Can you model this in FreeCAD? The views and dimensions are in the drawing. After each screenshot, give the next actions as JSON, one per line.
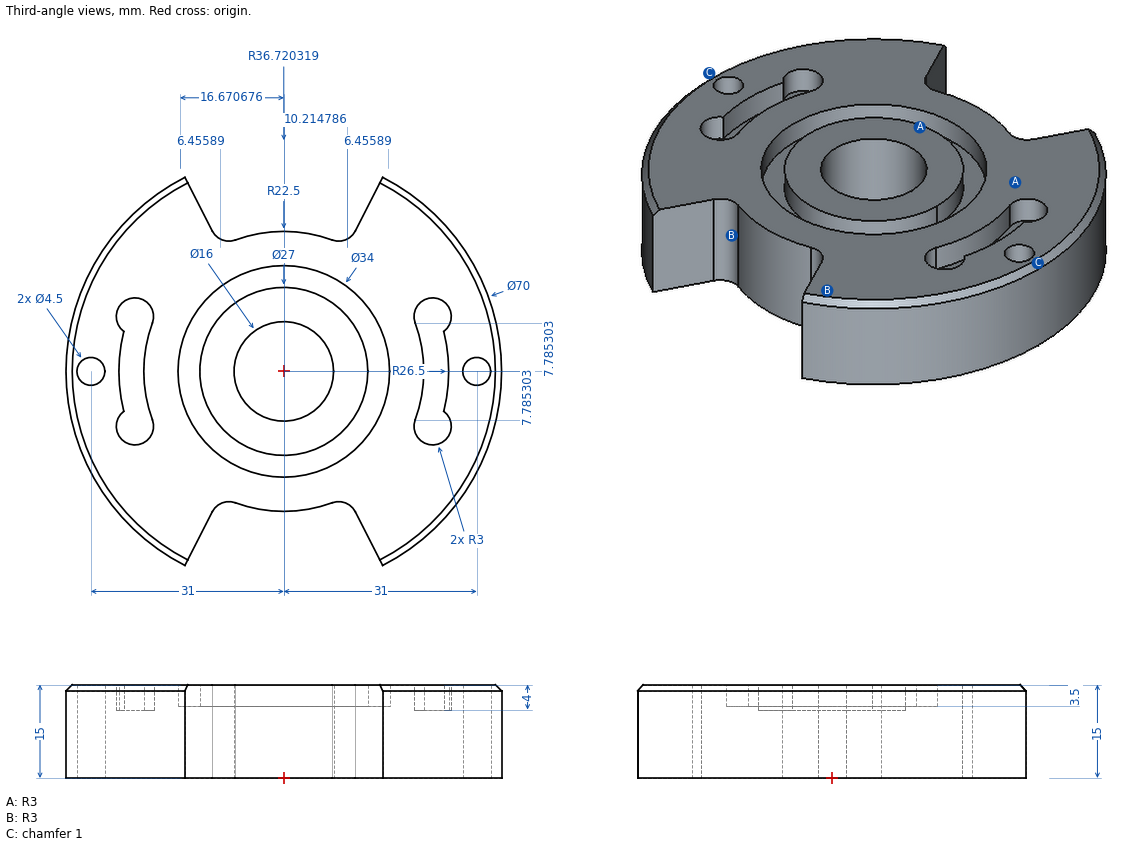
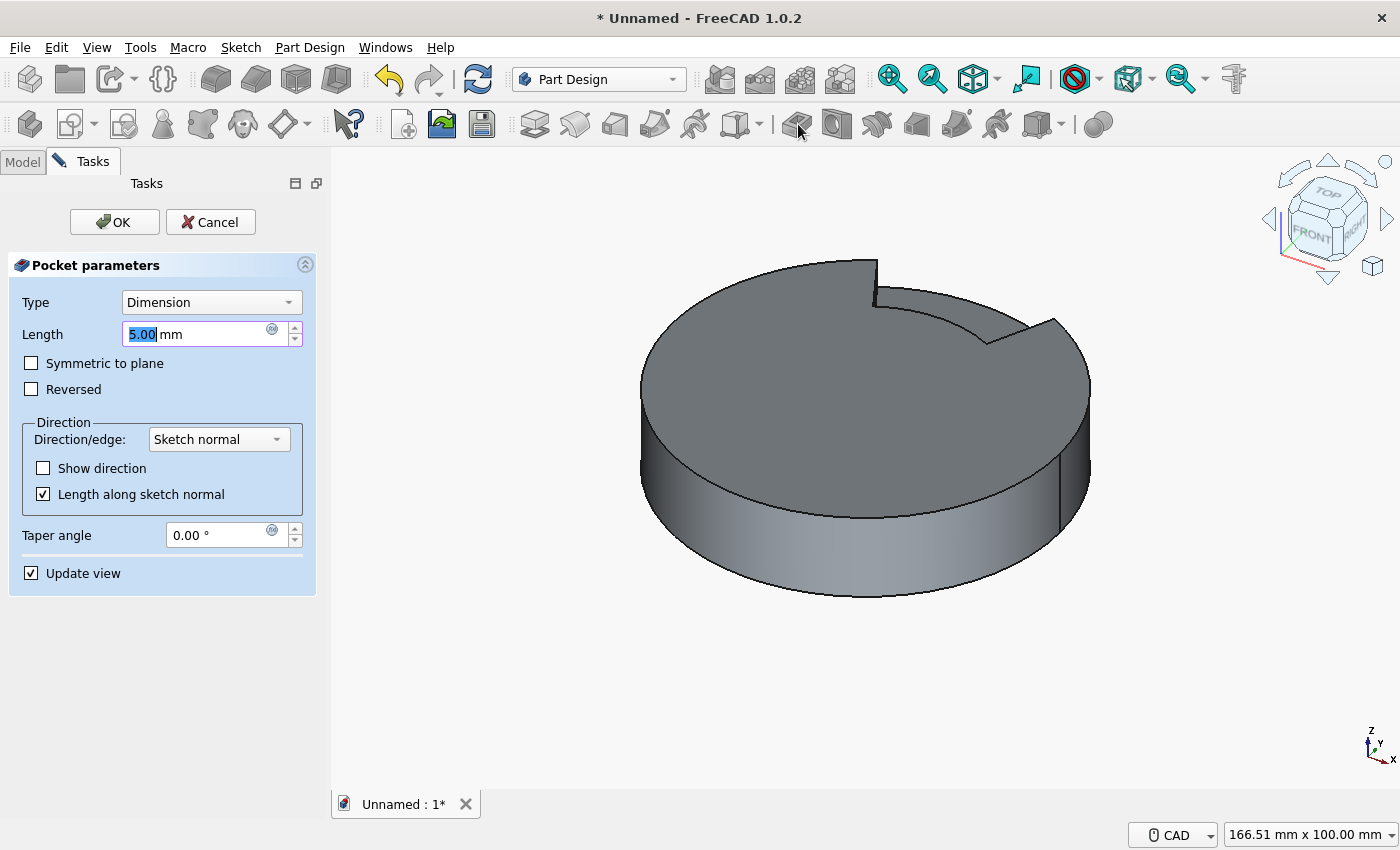
{"action": "type", "text": "15"}
{"action": "key", "text": "Tab"}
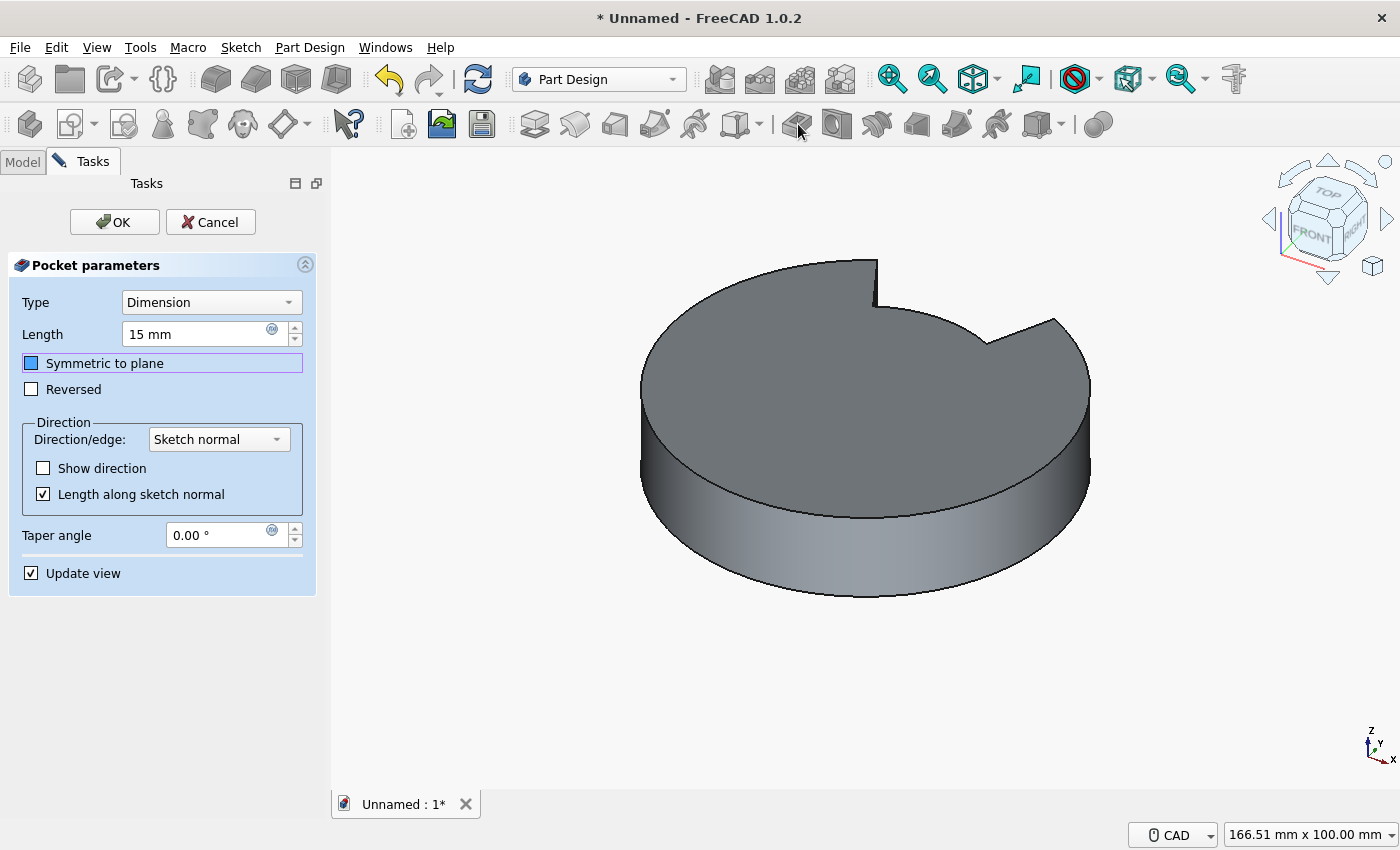
{"action": "left_click", "coordinate": [115, 222]}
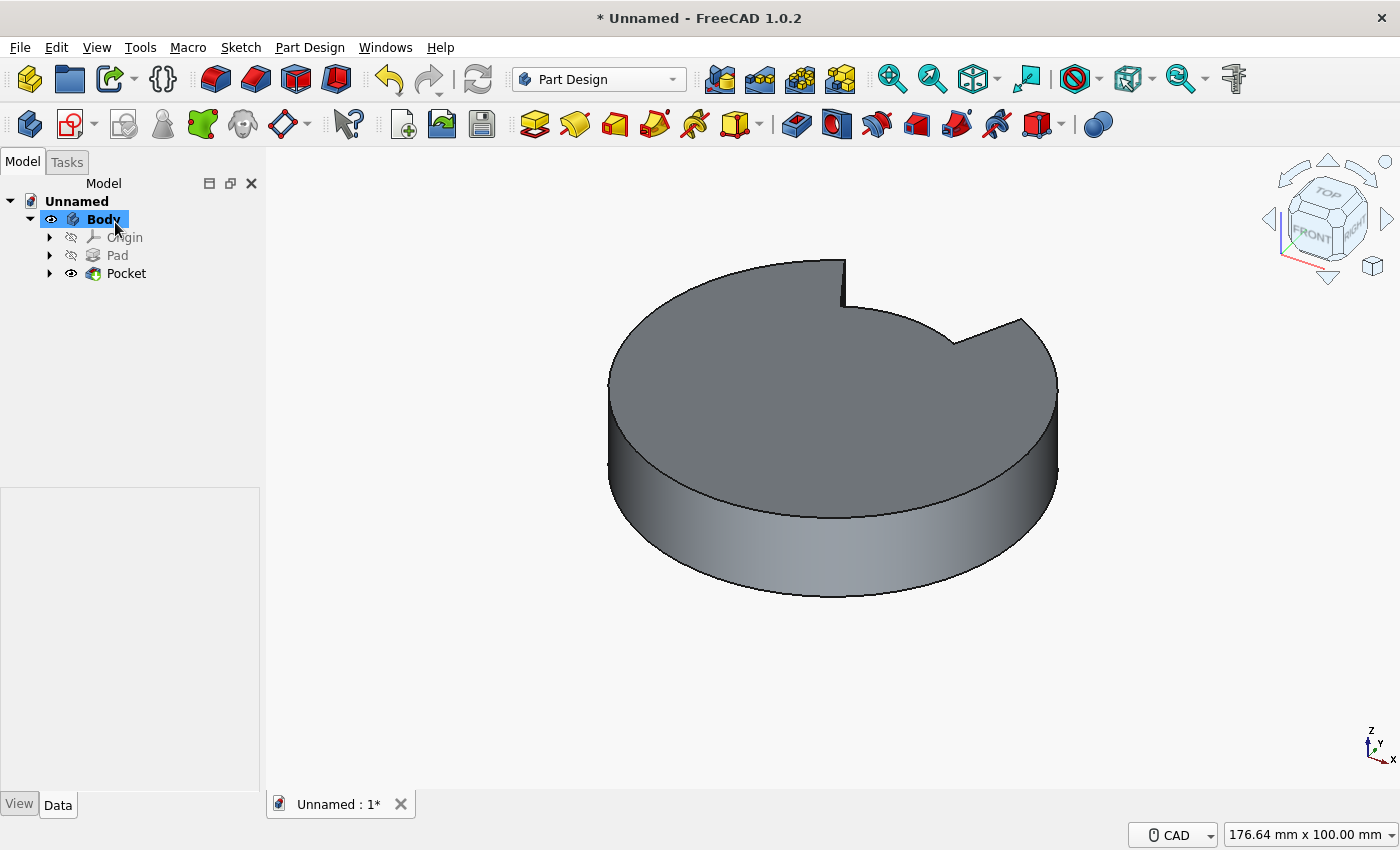
{"action": "key", "text": "0"}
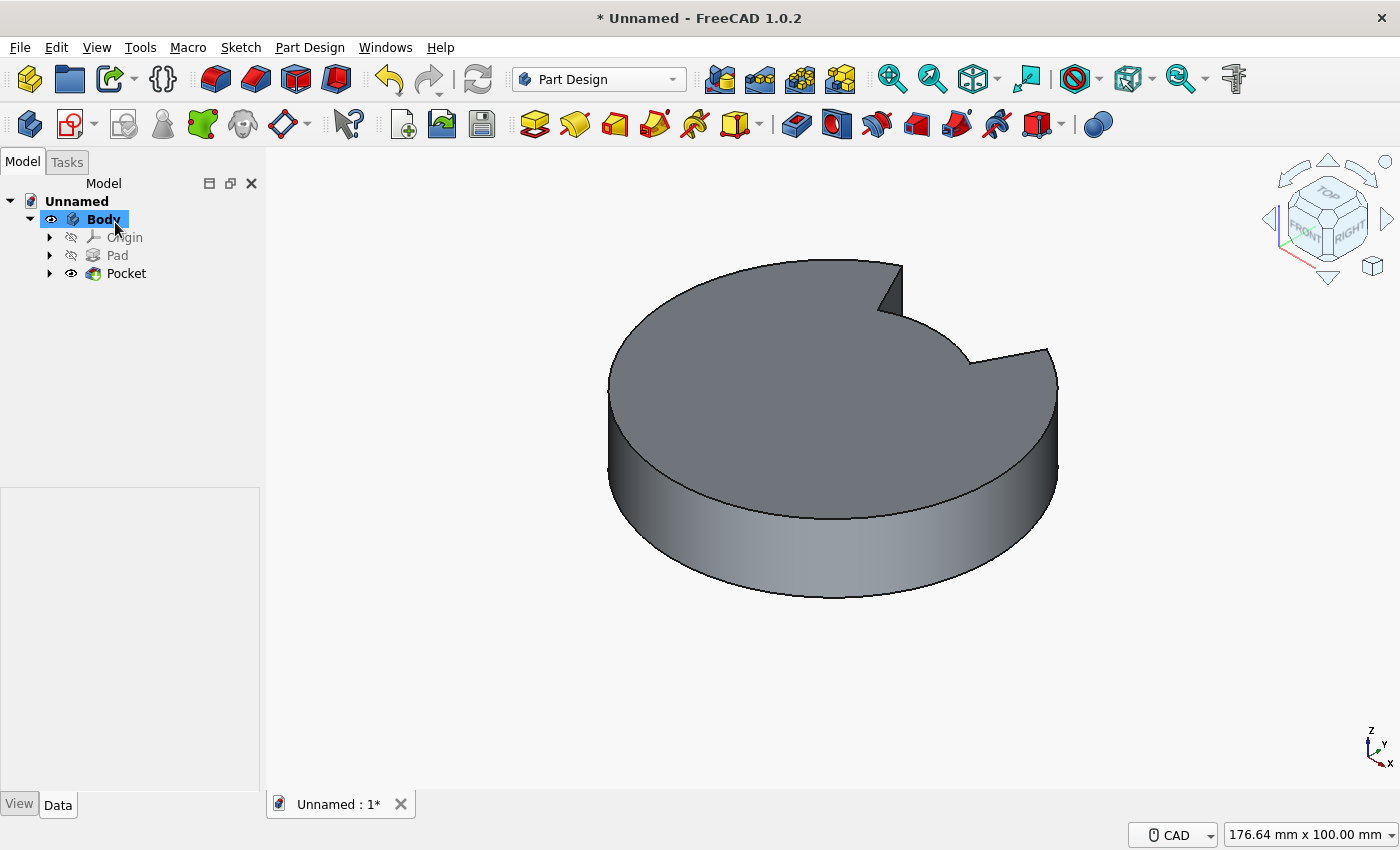
{"action": "key", "text": "2"}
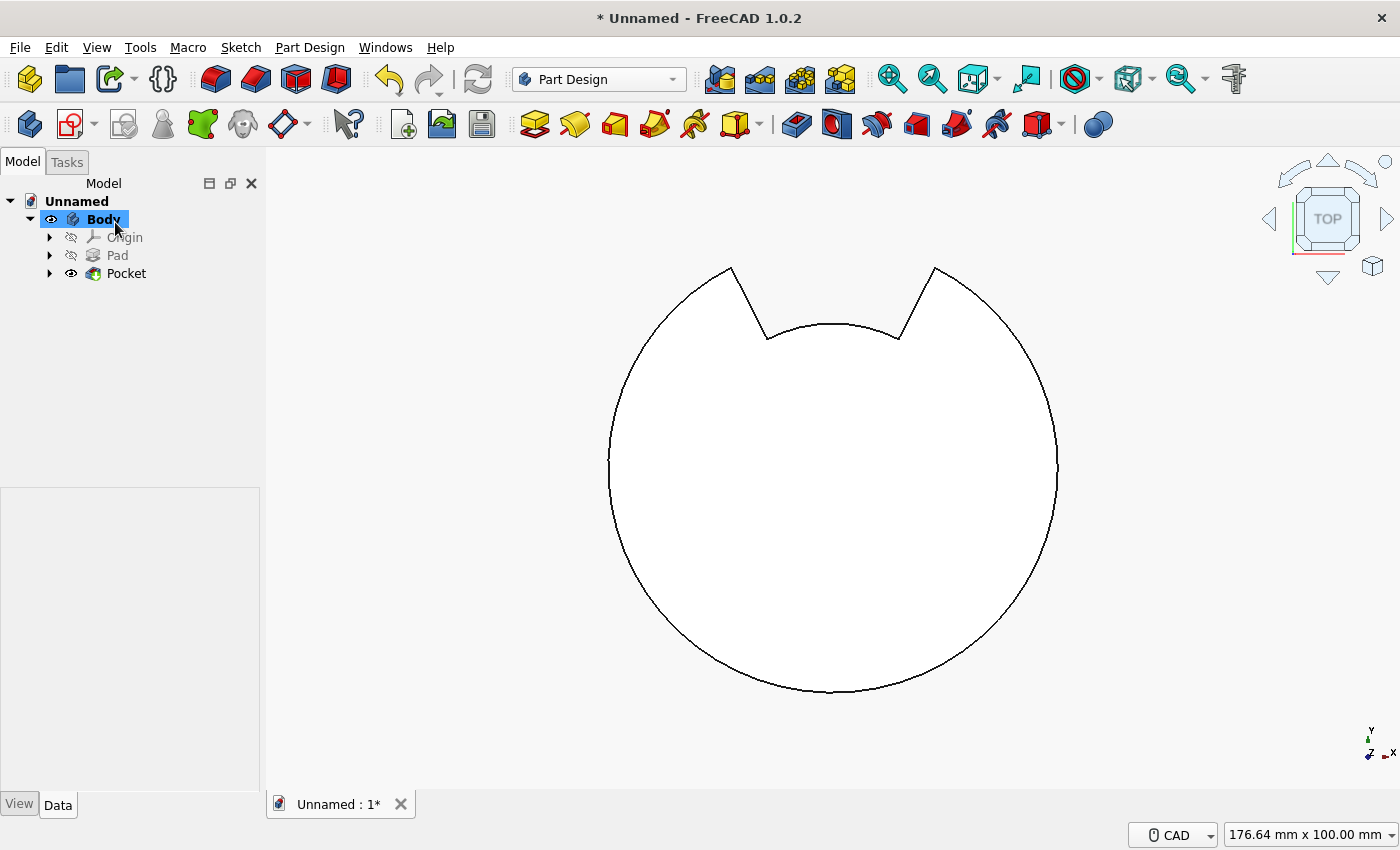
{"action": "key", "text": "1"}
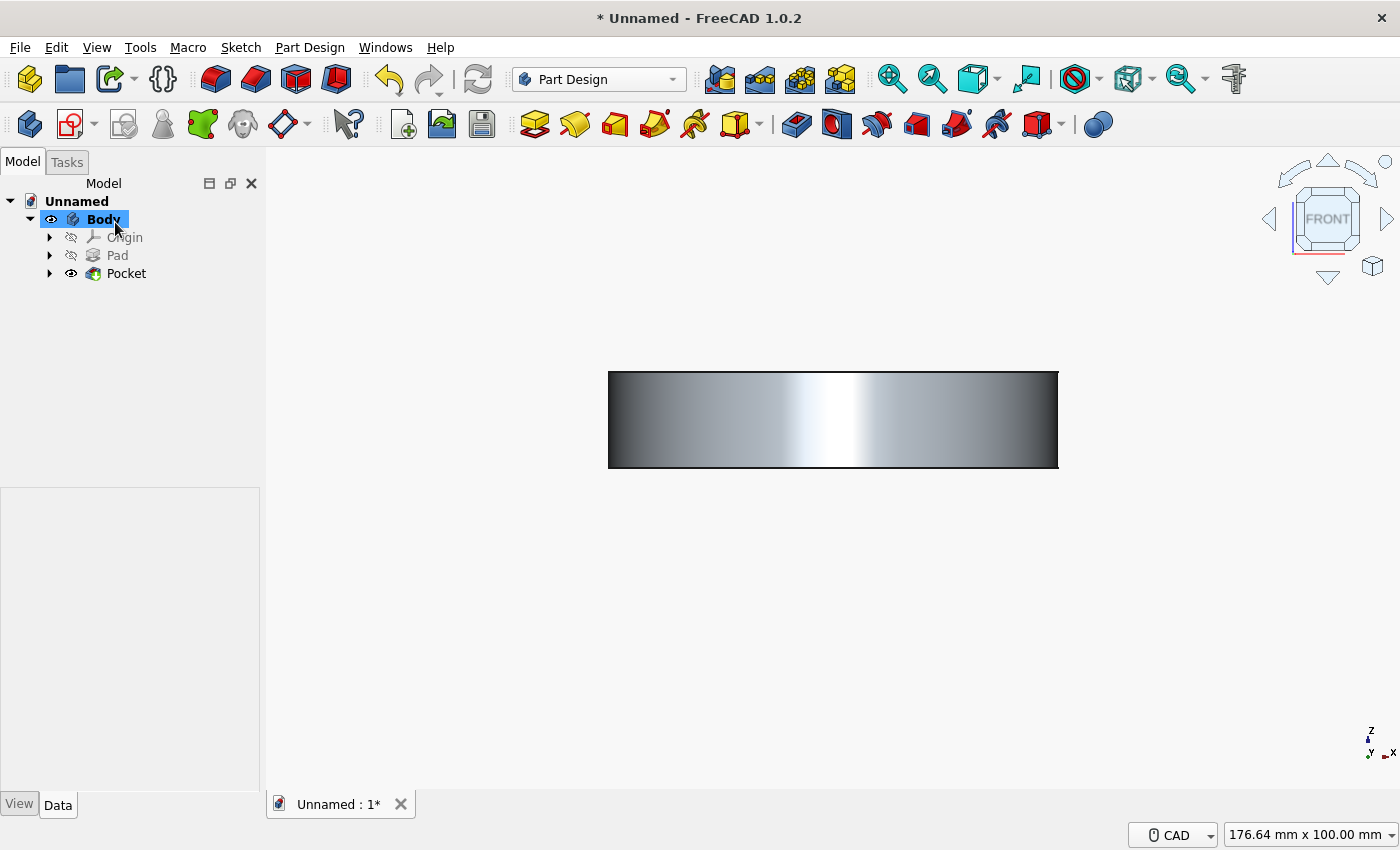
{"action": "left_click", "coordinate": [894, 80]}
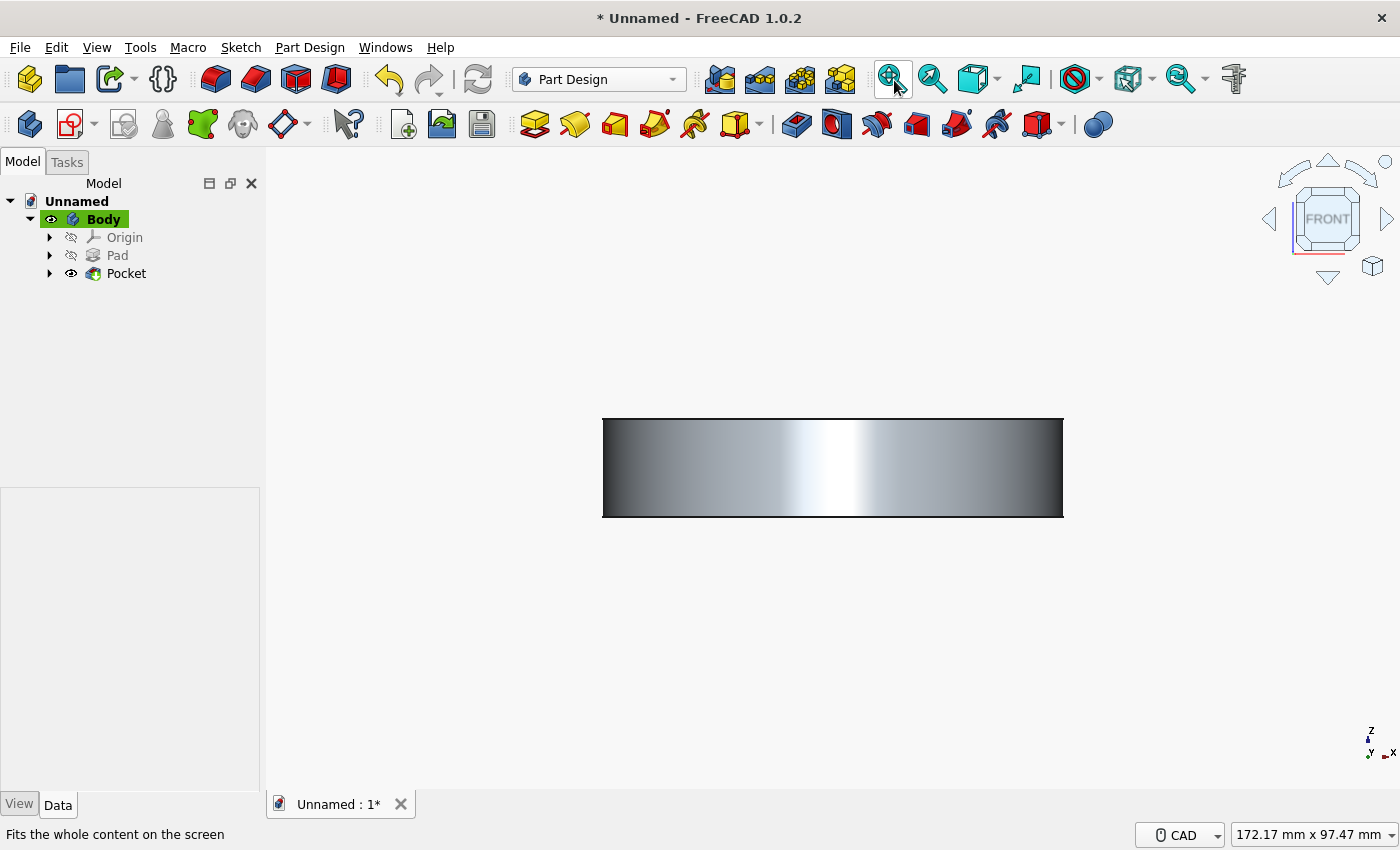
{"action": "key", "text": "3"}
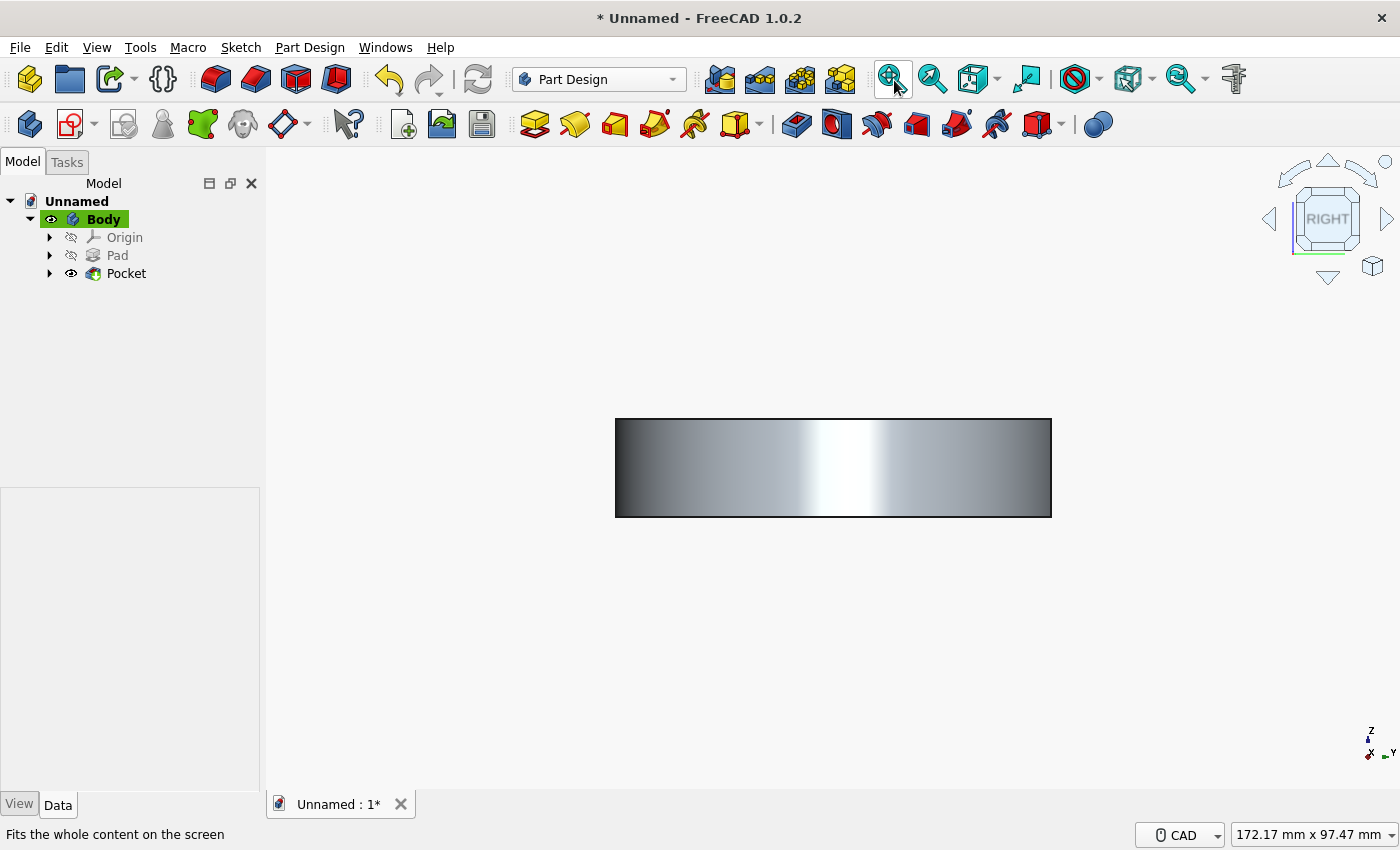
{"action": "left_click", "coordinate": [894, 80]}